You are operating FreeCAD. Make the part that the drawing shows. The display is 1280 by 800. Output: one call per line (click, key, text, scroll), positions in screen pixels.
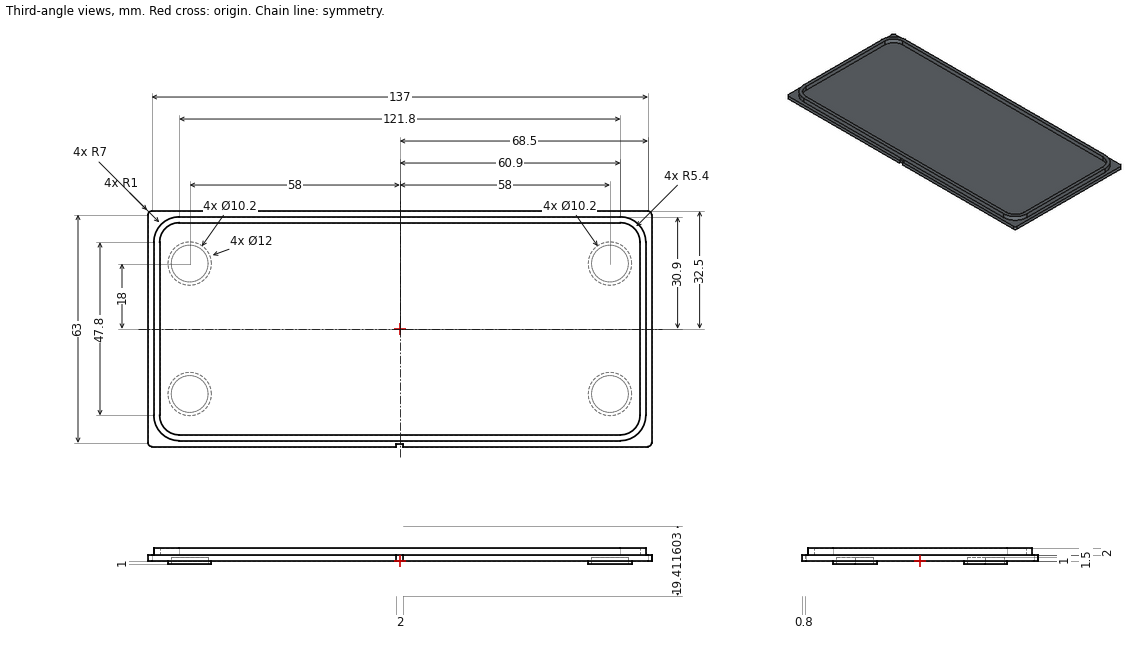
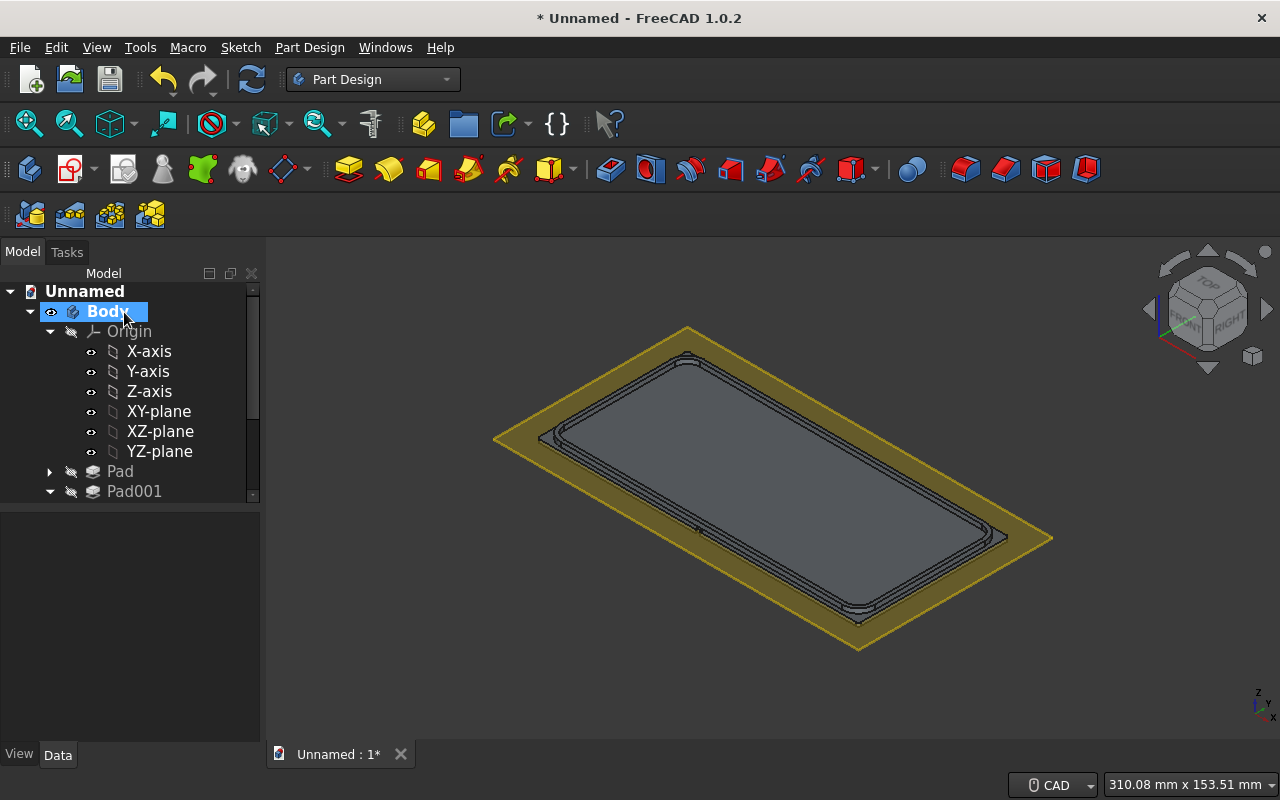
scroll(100, 387, down, 3)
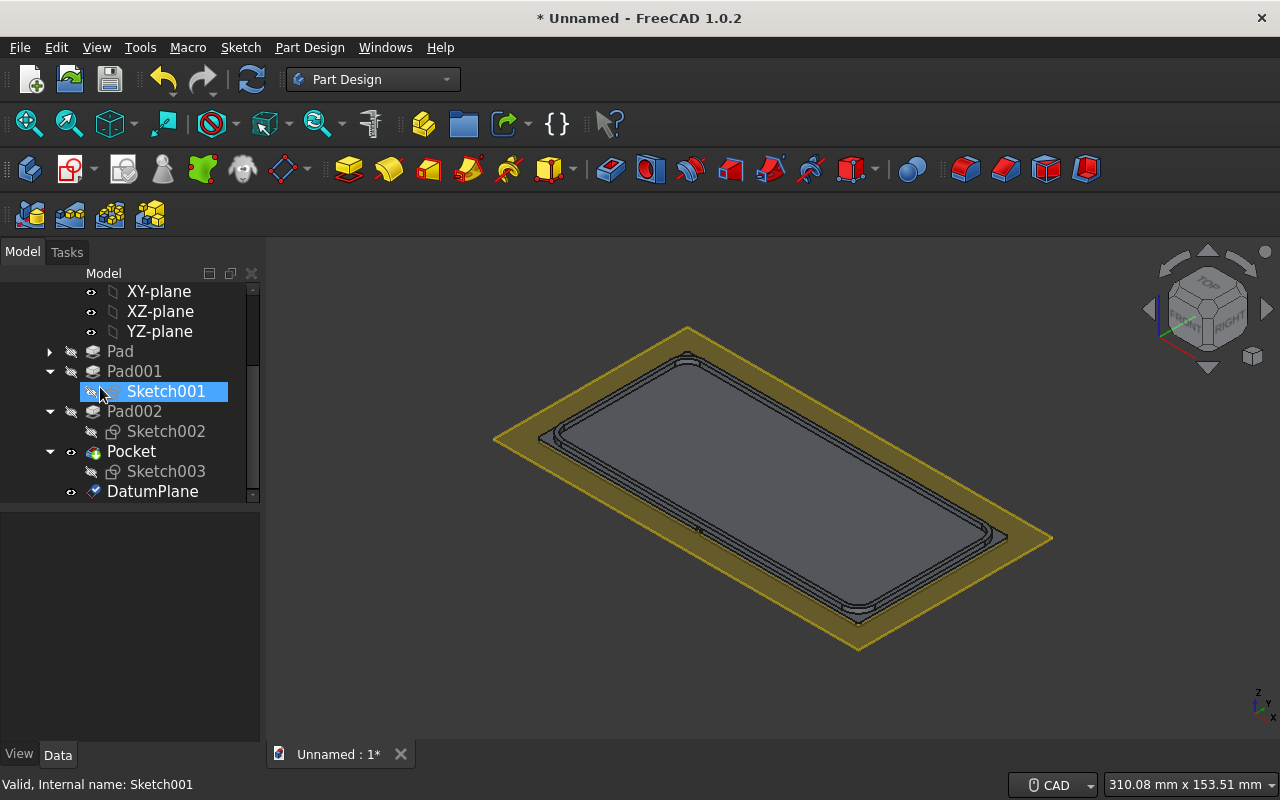
click(116, 492)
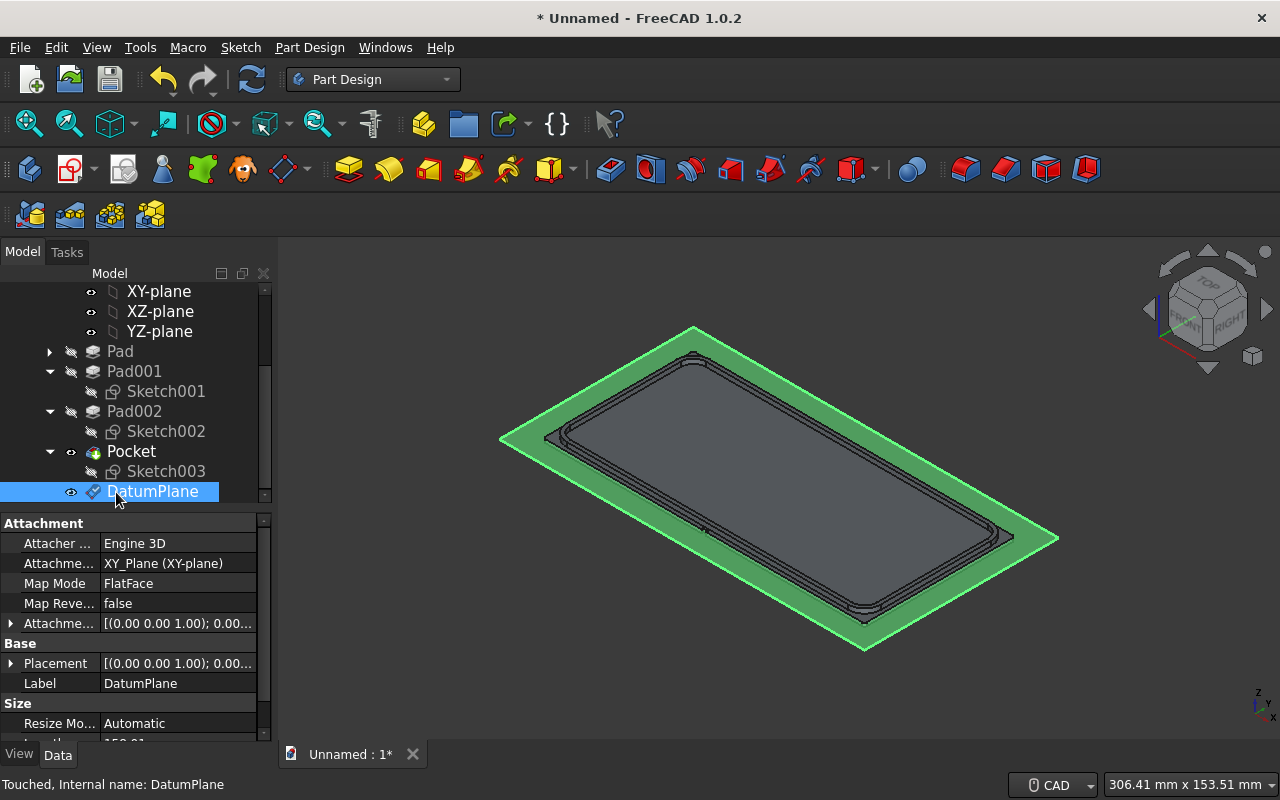
click(70, 170)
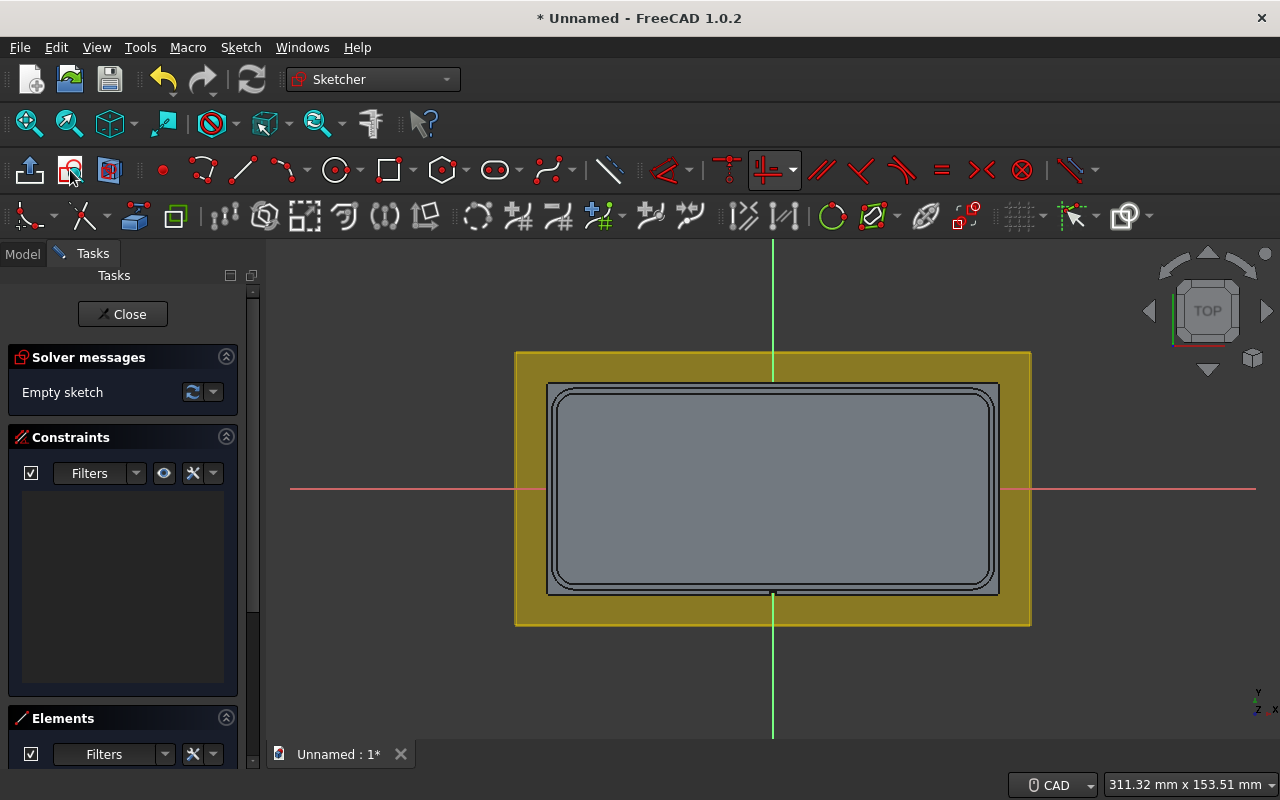
click(110, 170)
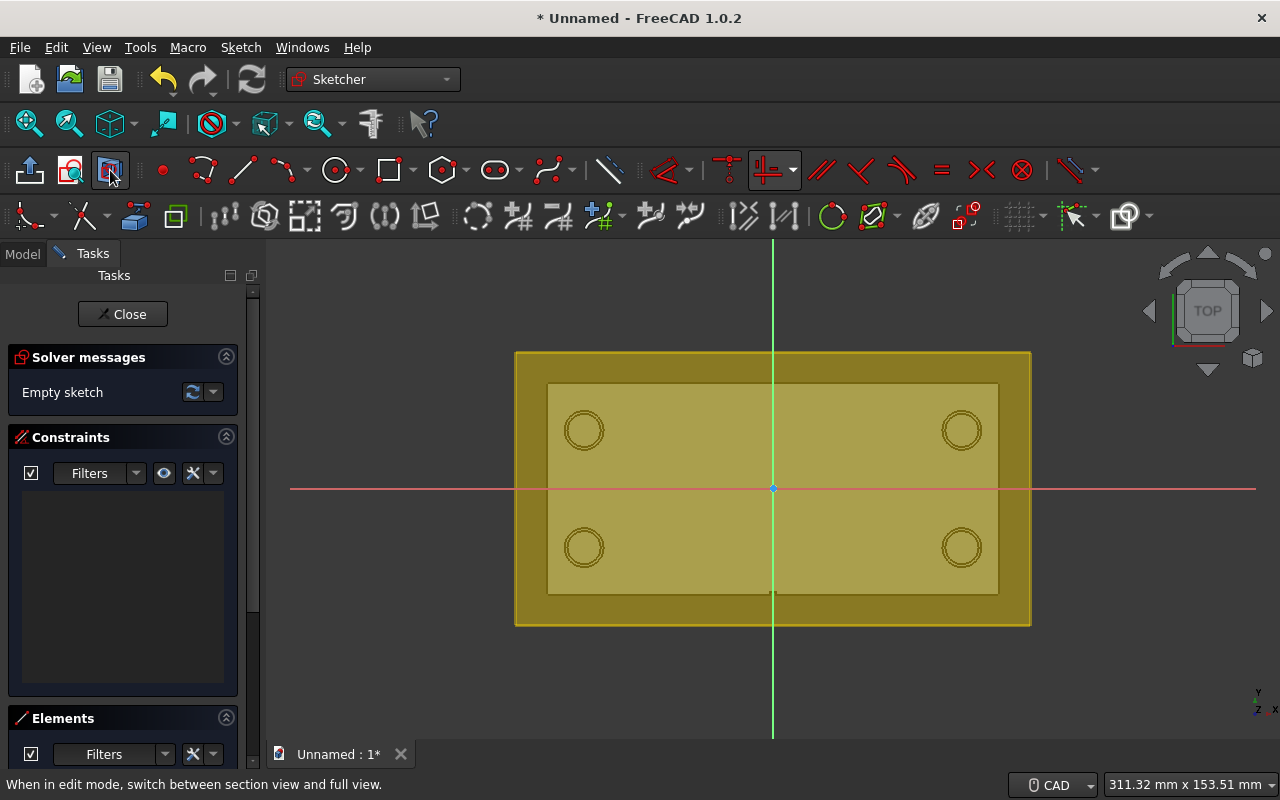
scroll(912, 489, up, 2)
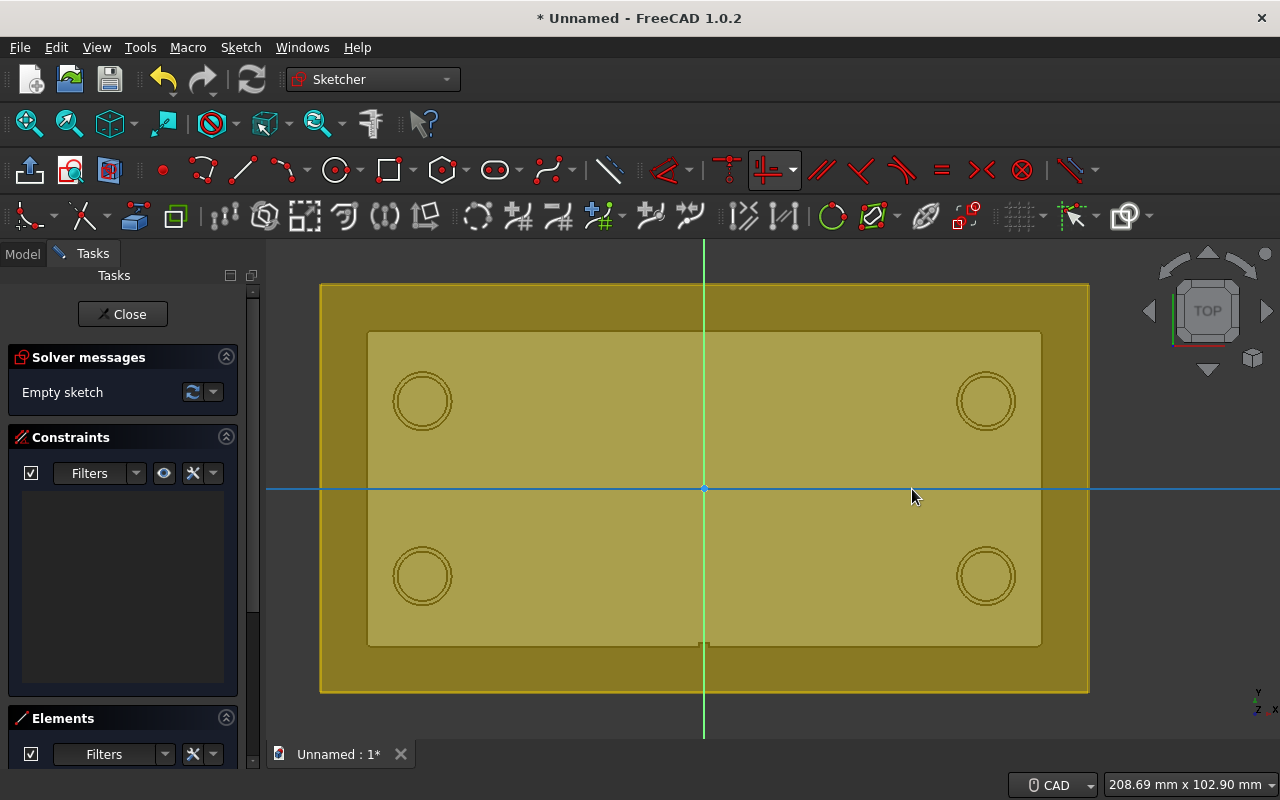
click(336, 170)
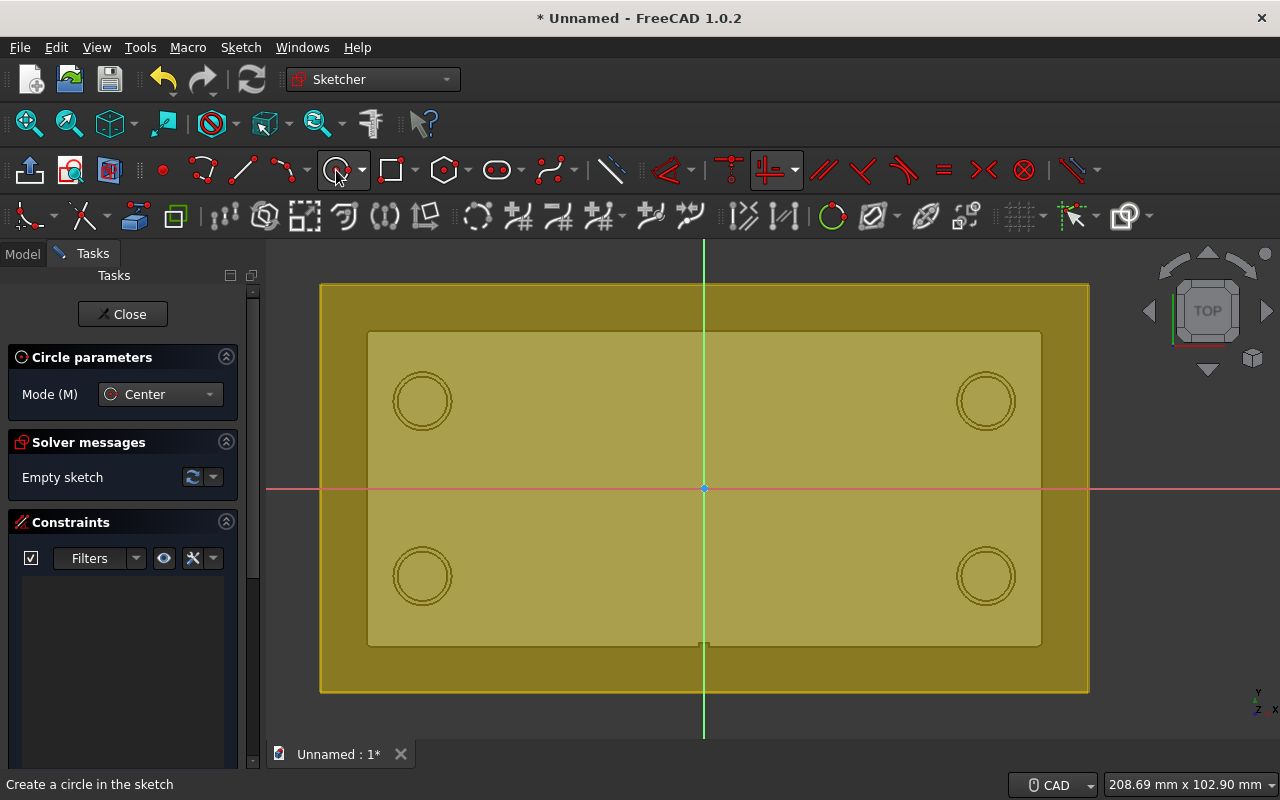
click(986, 401)
move(1004, 384)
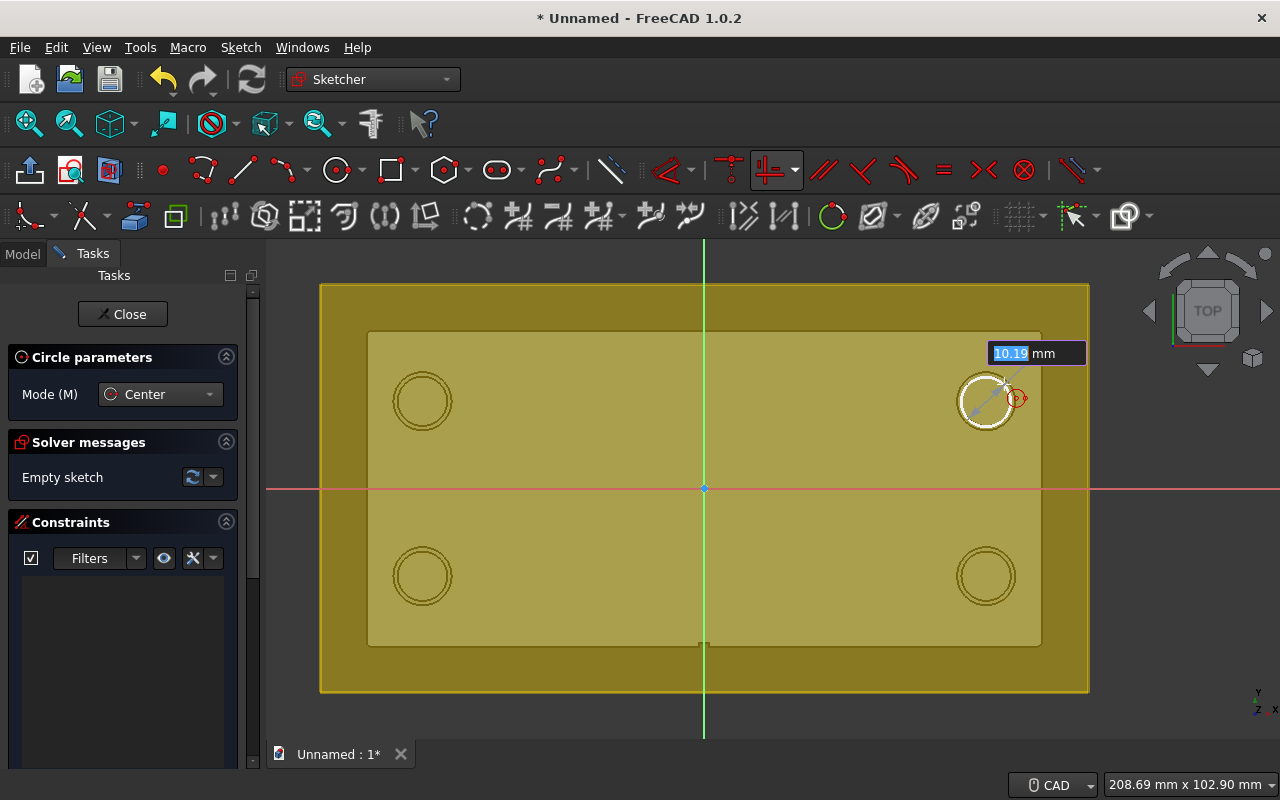
text(10.2)
key(Return)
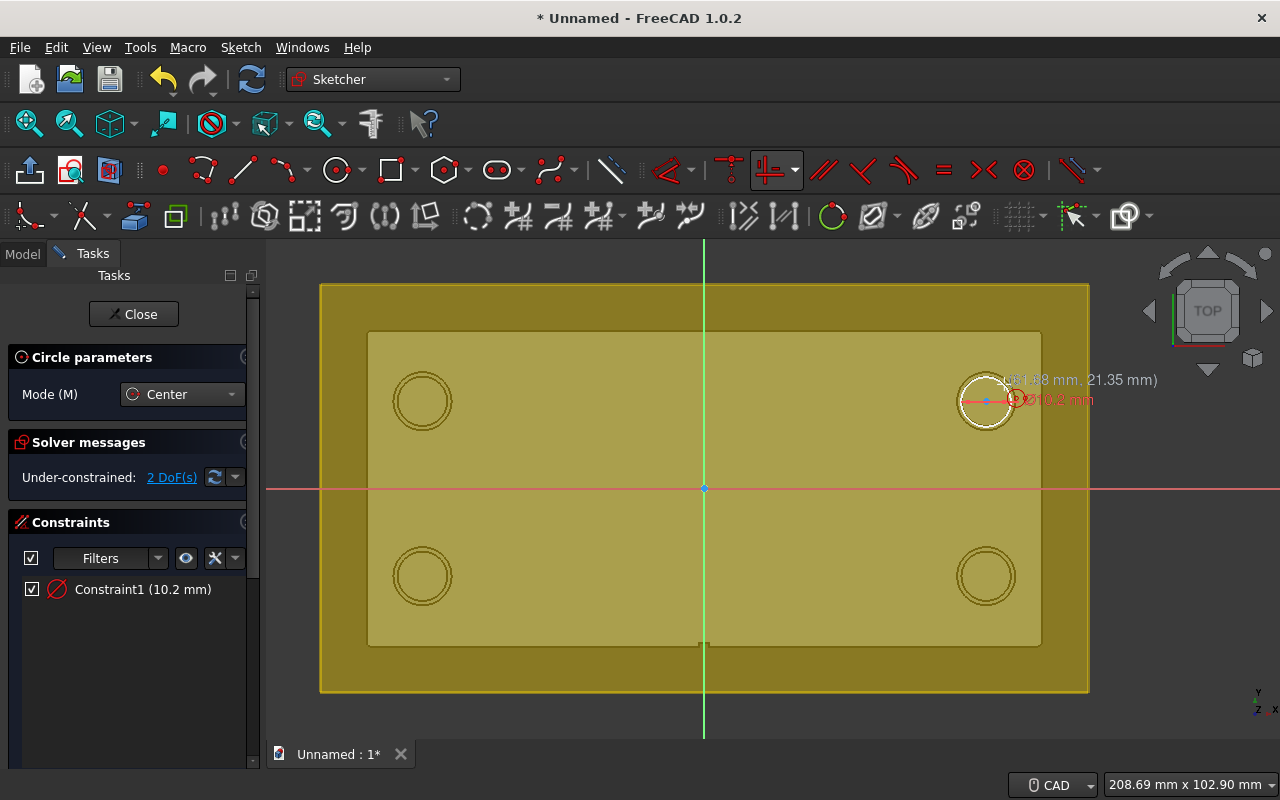
click(423, 401)
move(440, 384)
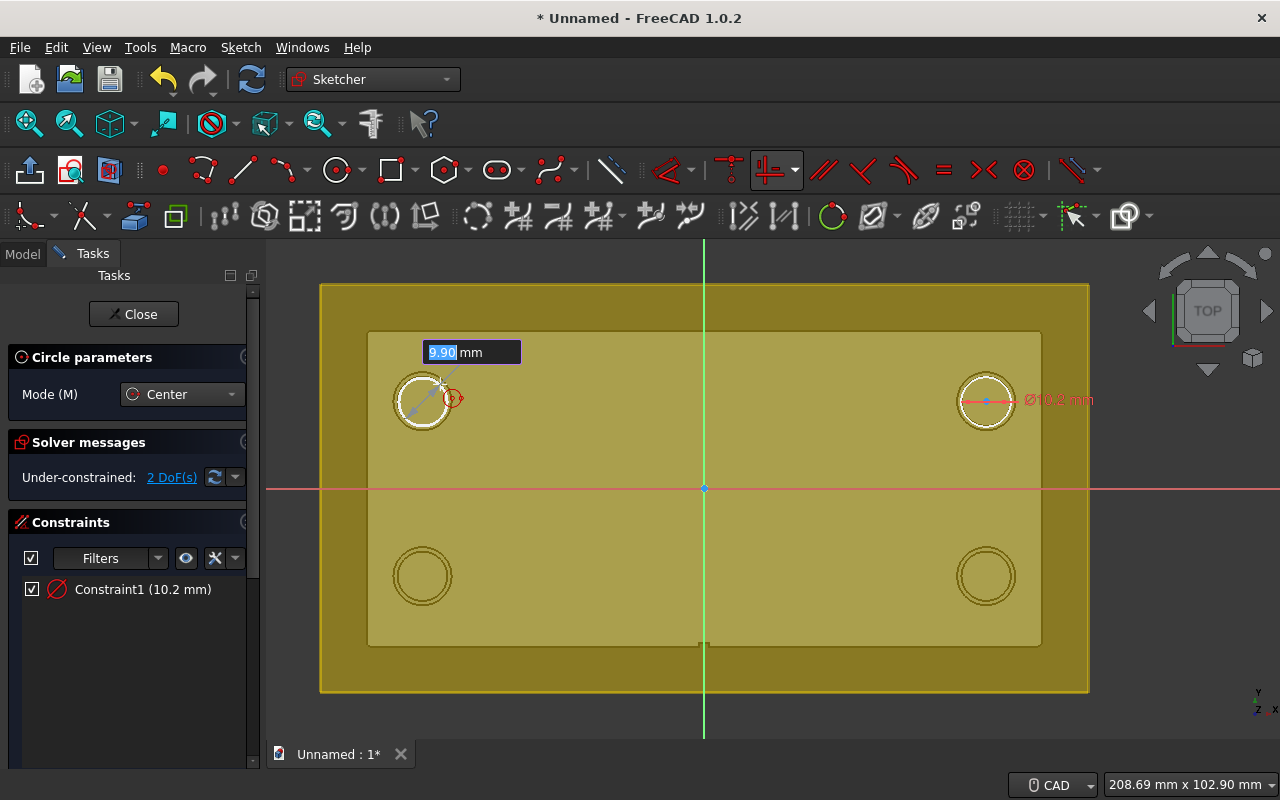
text(10.2)
key(Return)